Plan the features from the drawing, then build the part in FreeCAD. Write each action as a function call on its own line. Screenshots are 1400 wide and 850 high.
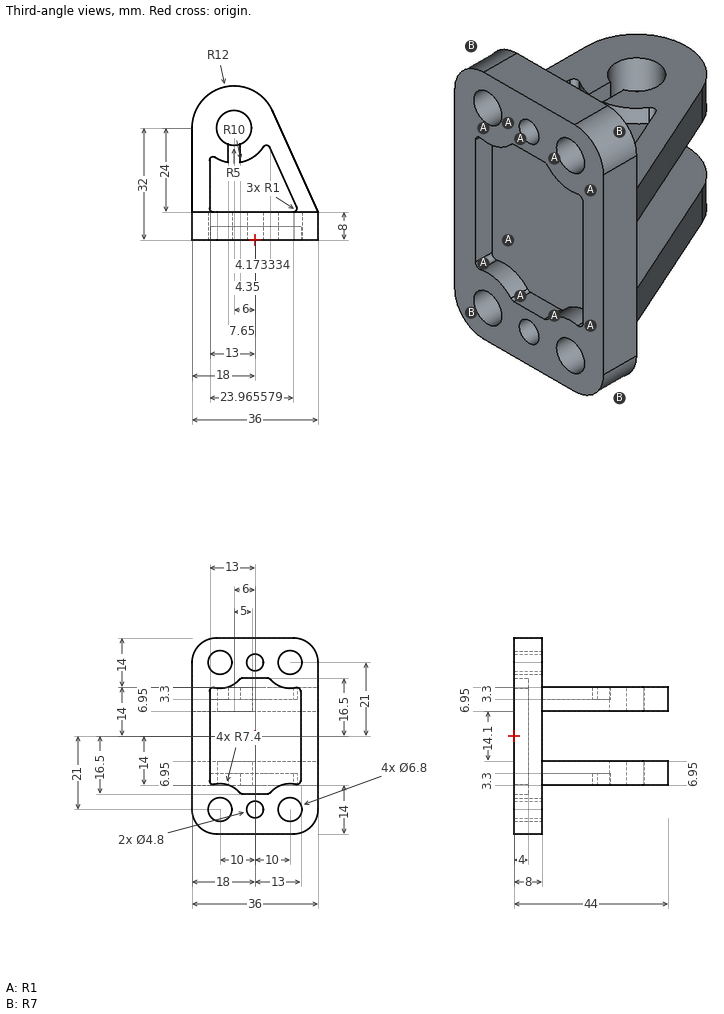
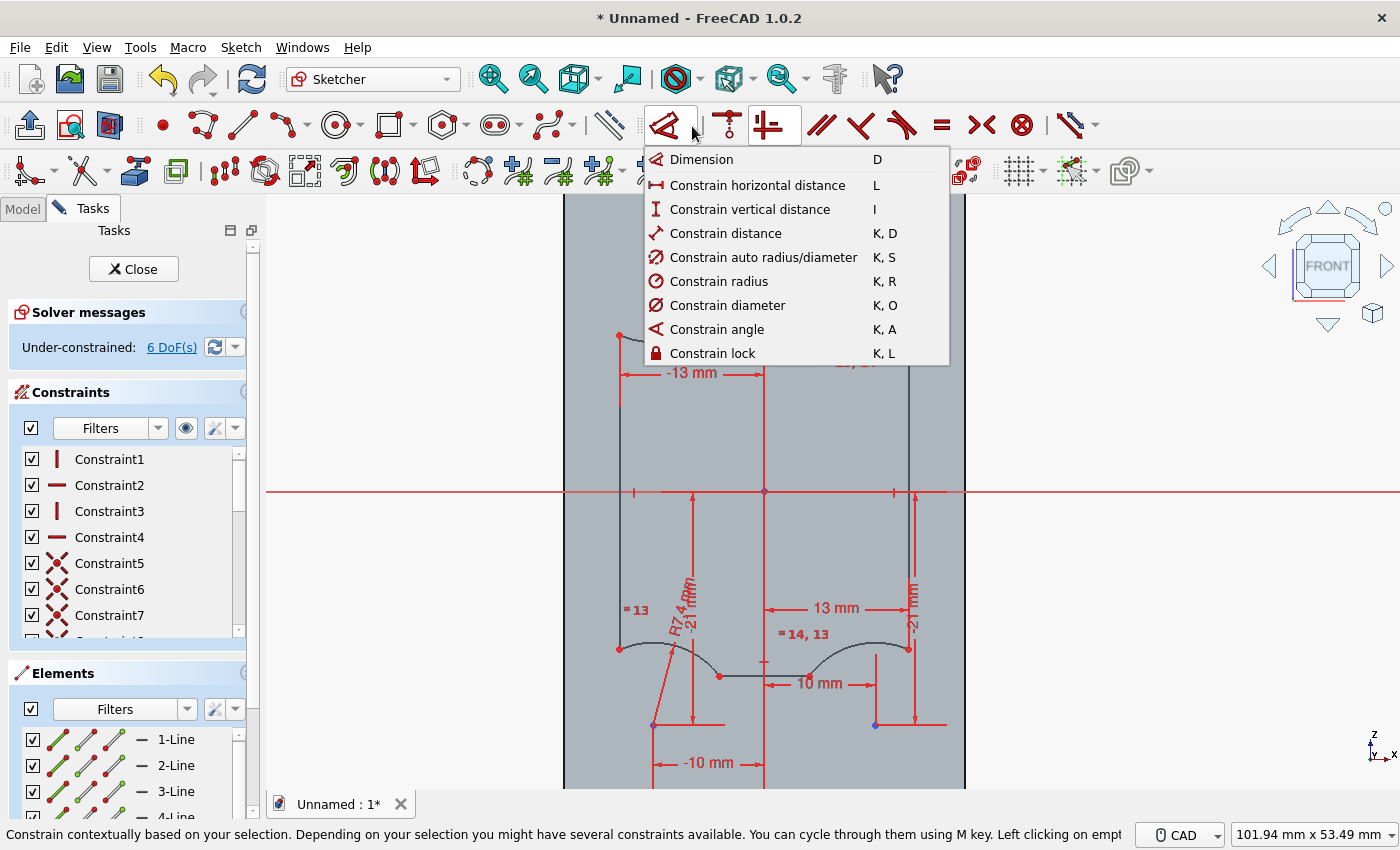
click(797, 185)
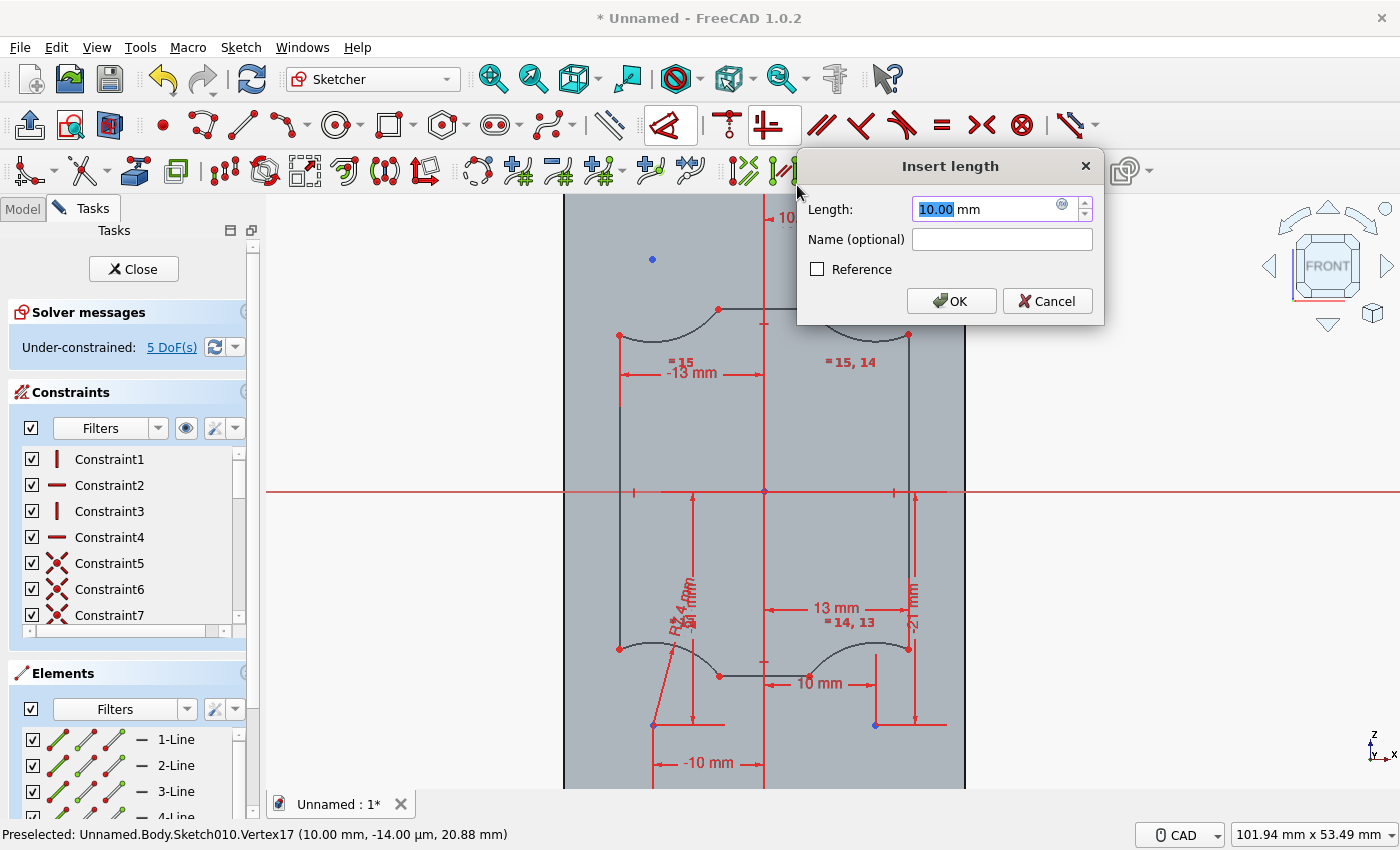
text(10)
key(Return)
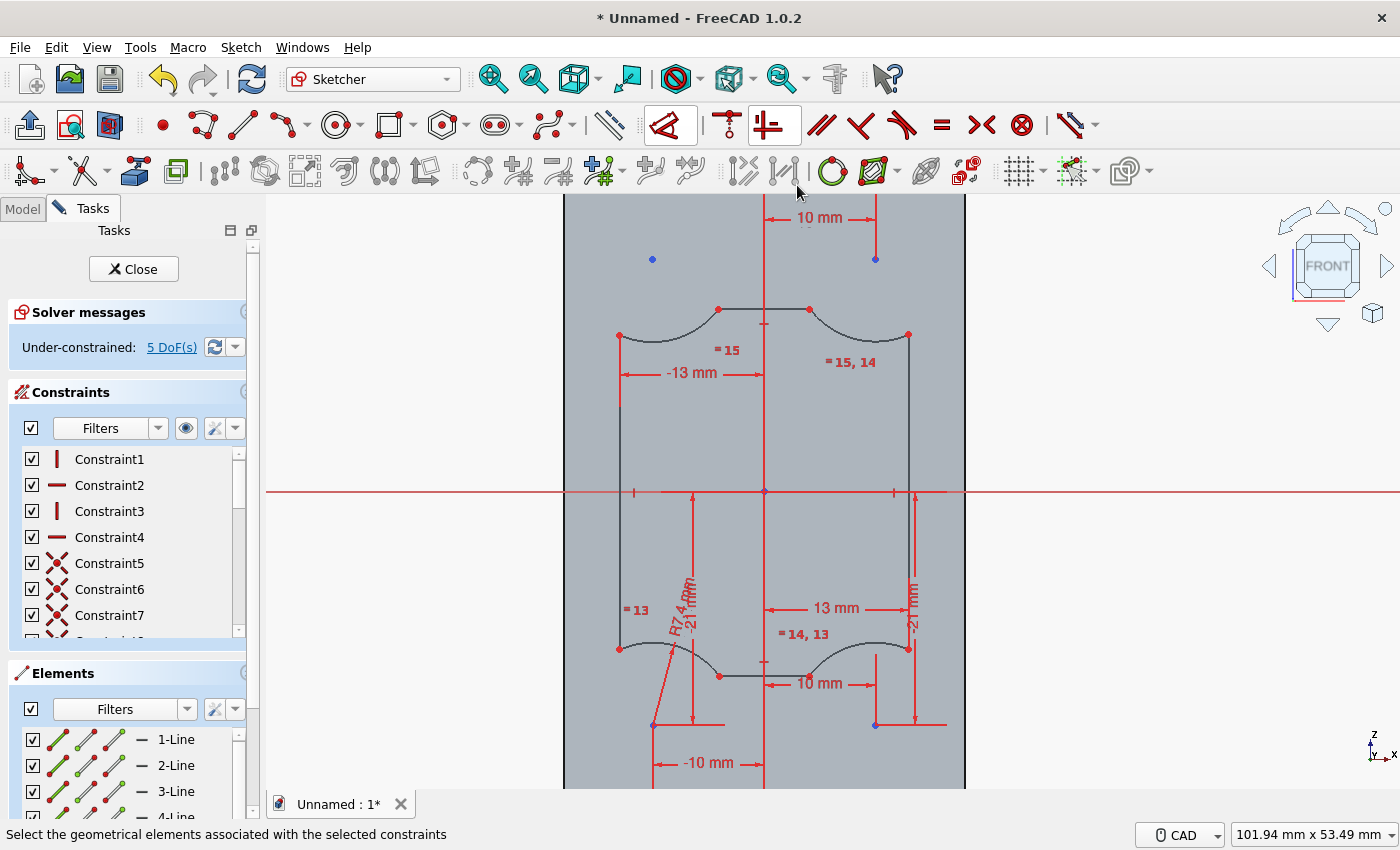
click(876, 259)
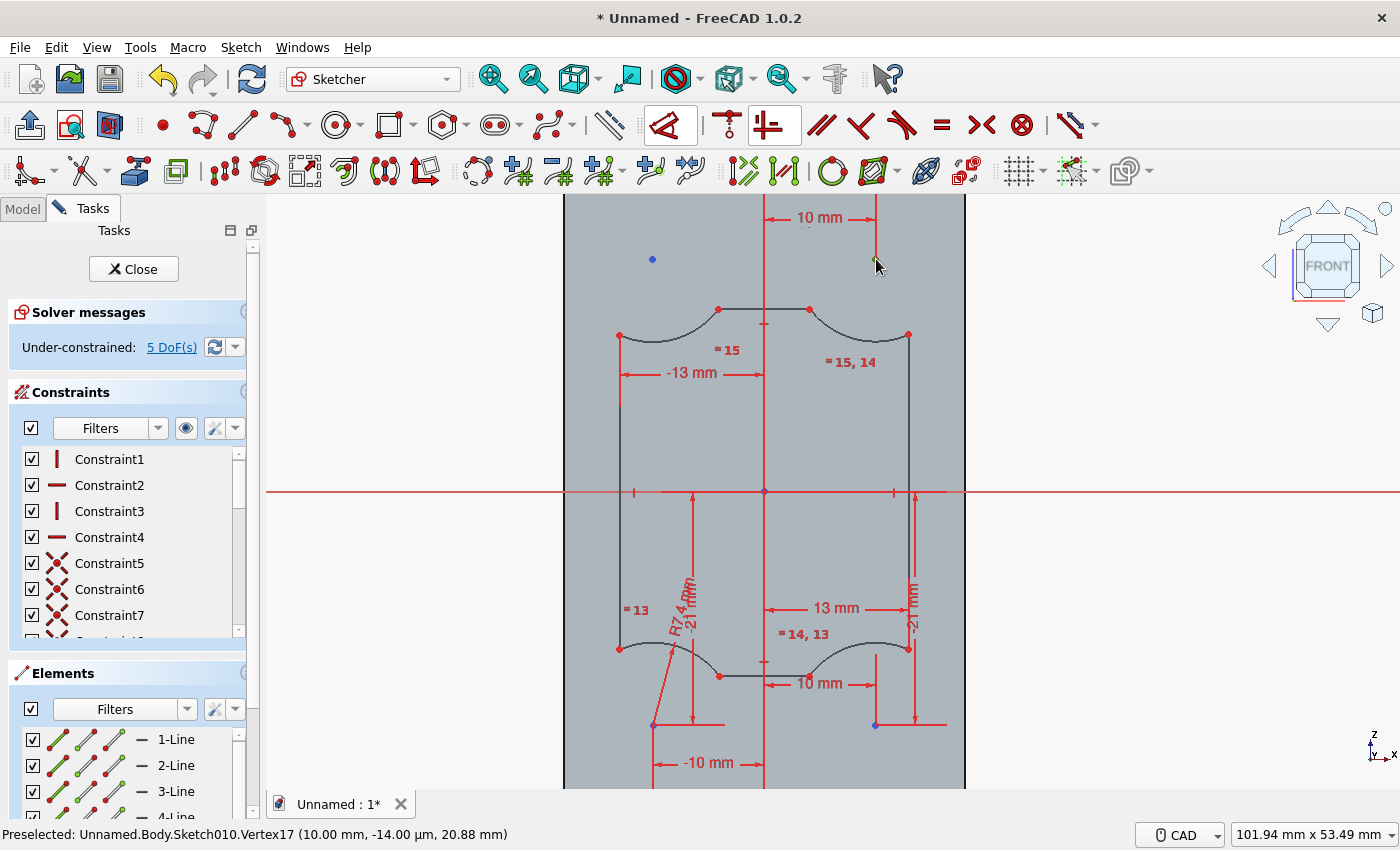
key(i)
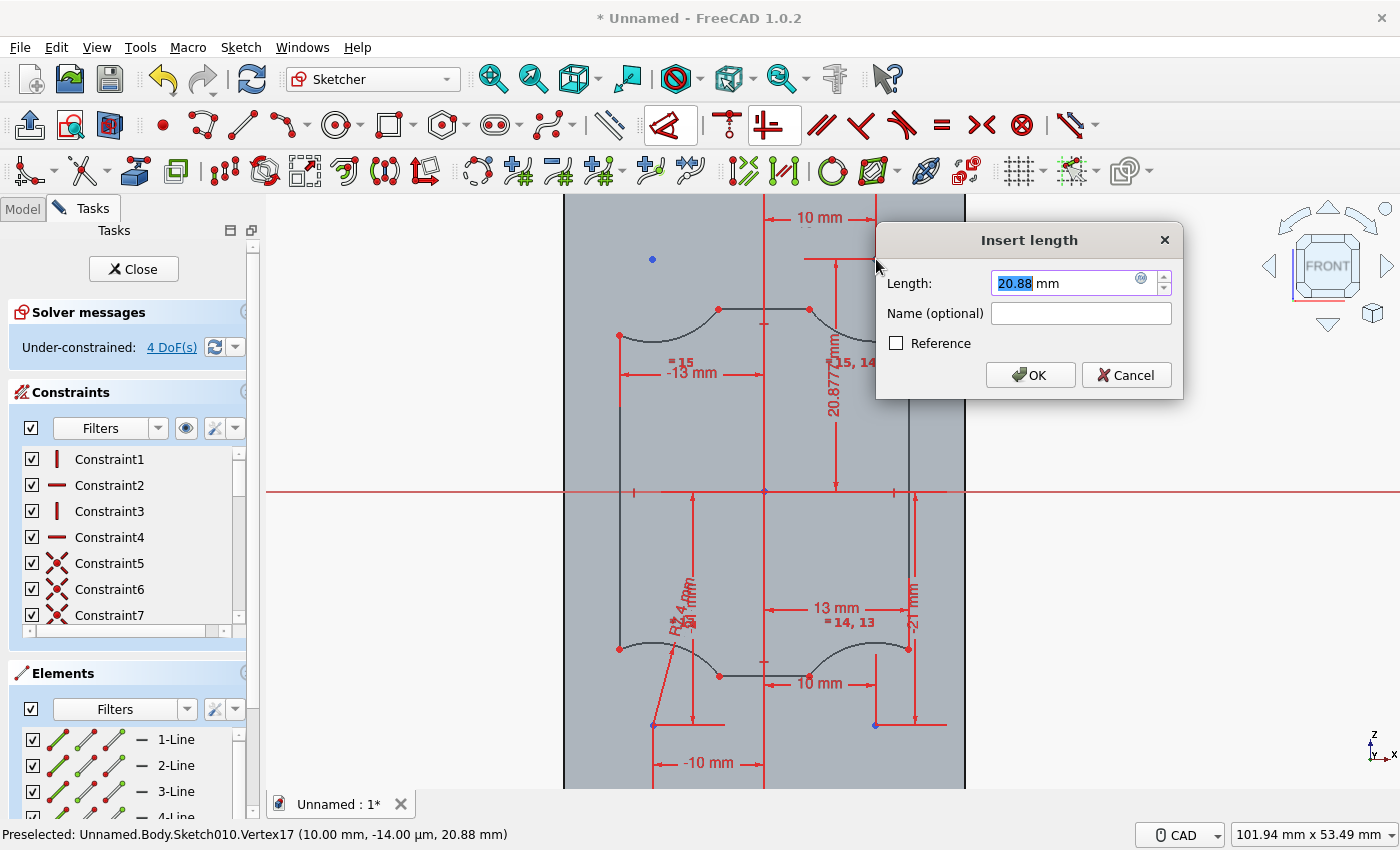
text(21)
key(Return)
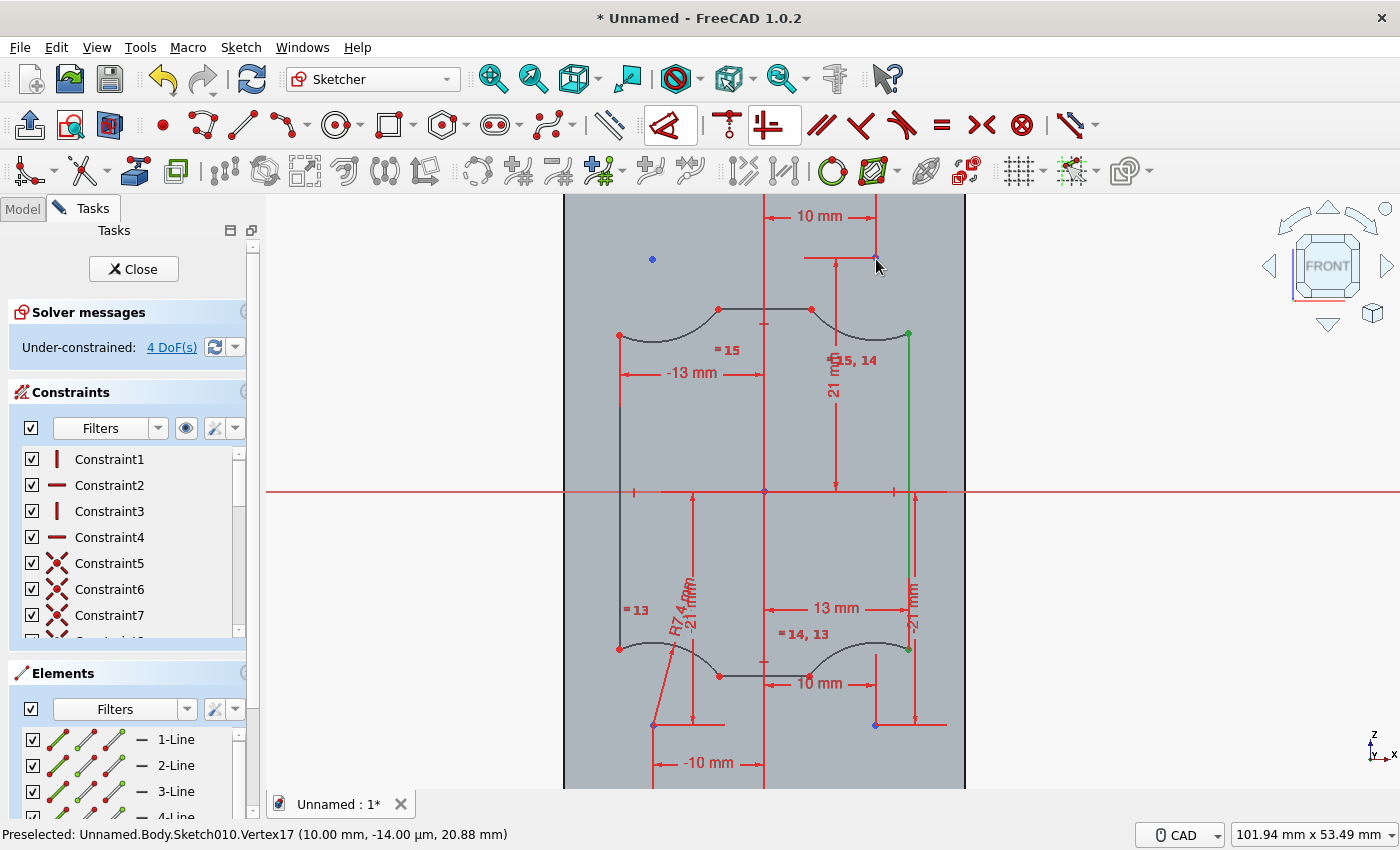
click(653, 260)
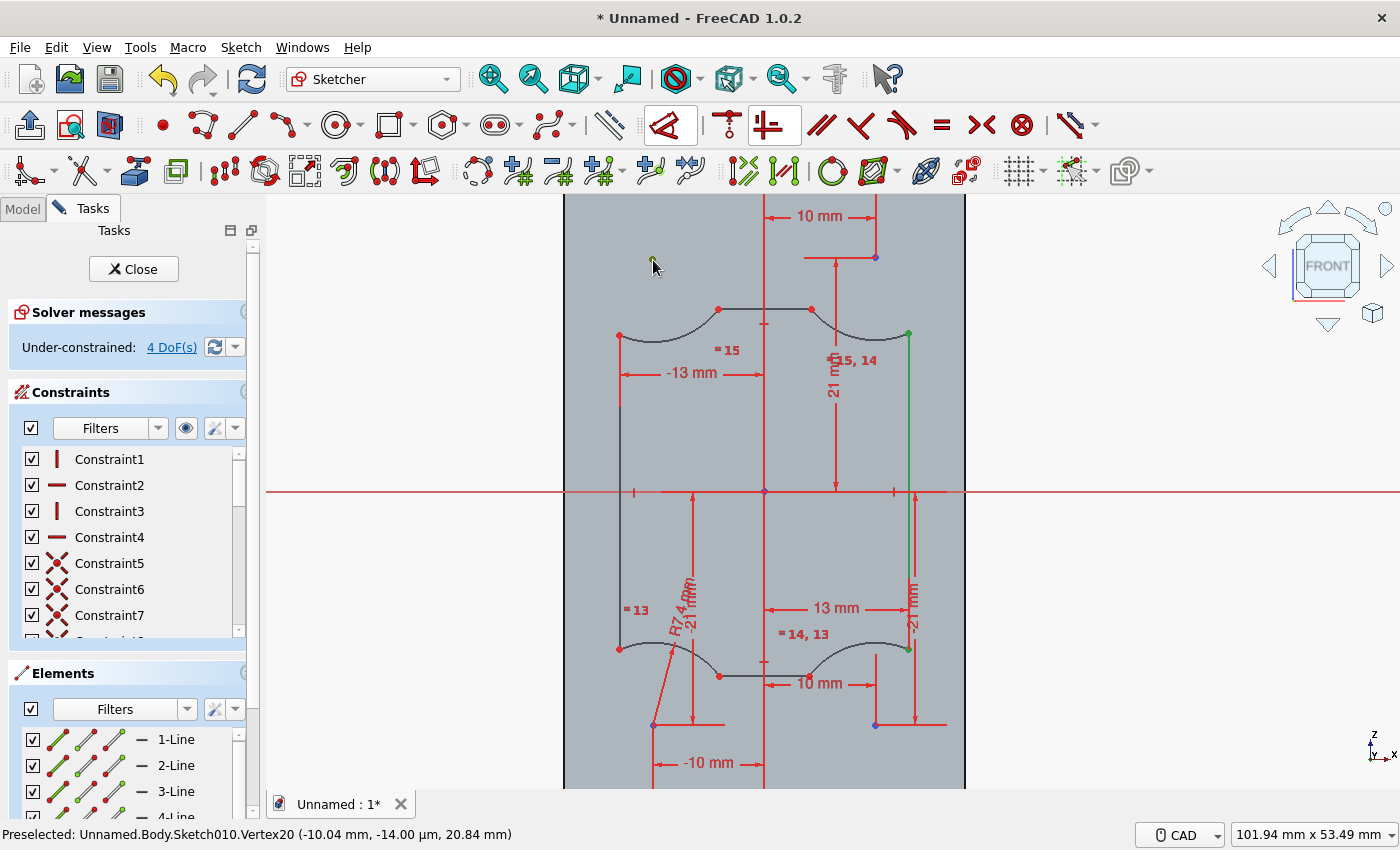
key(l)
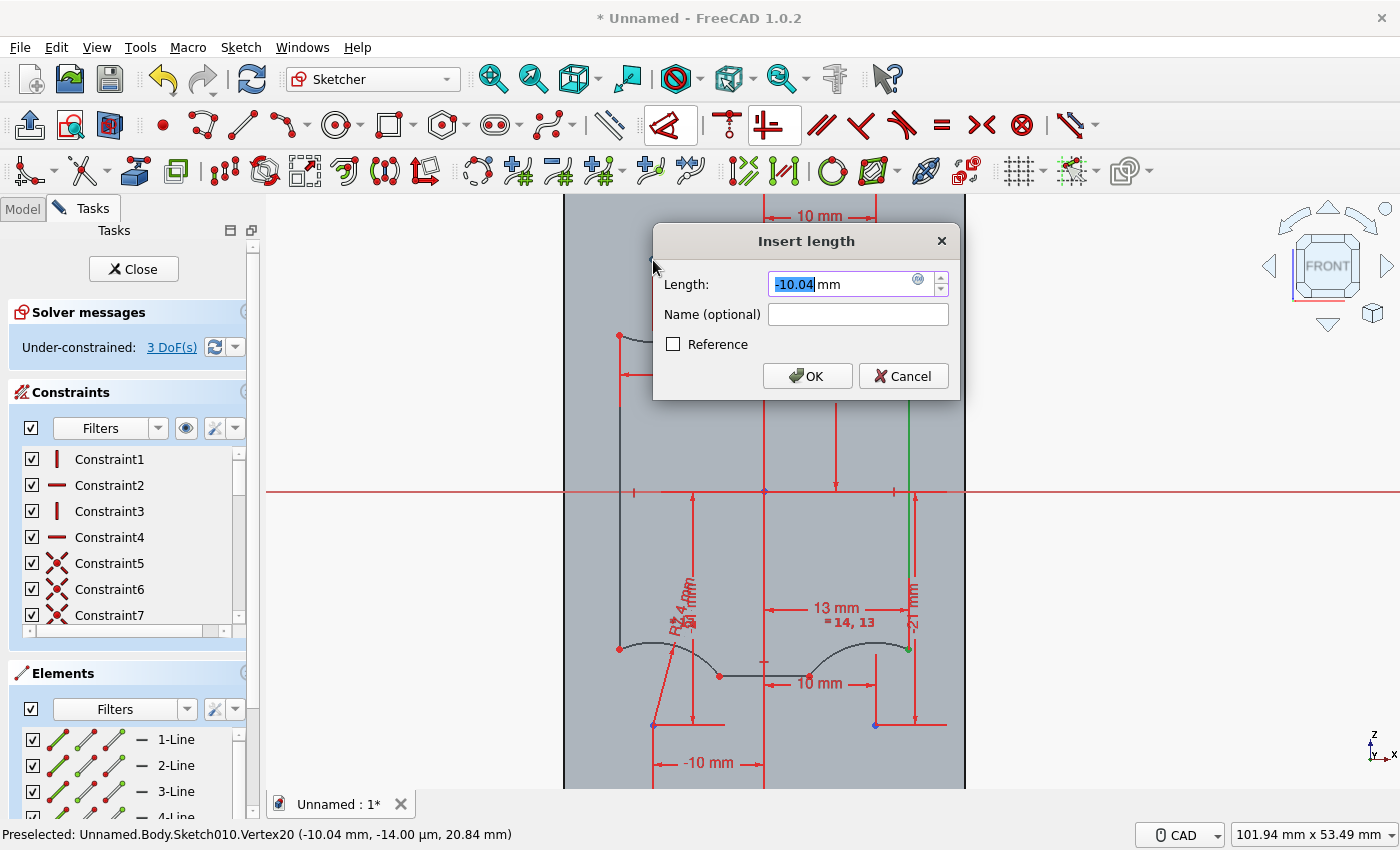
text(-10)
key(Return)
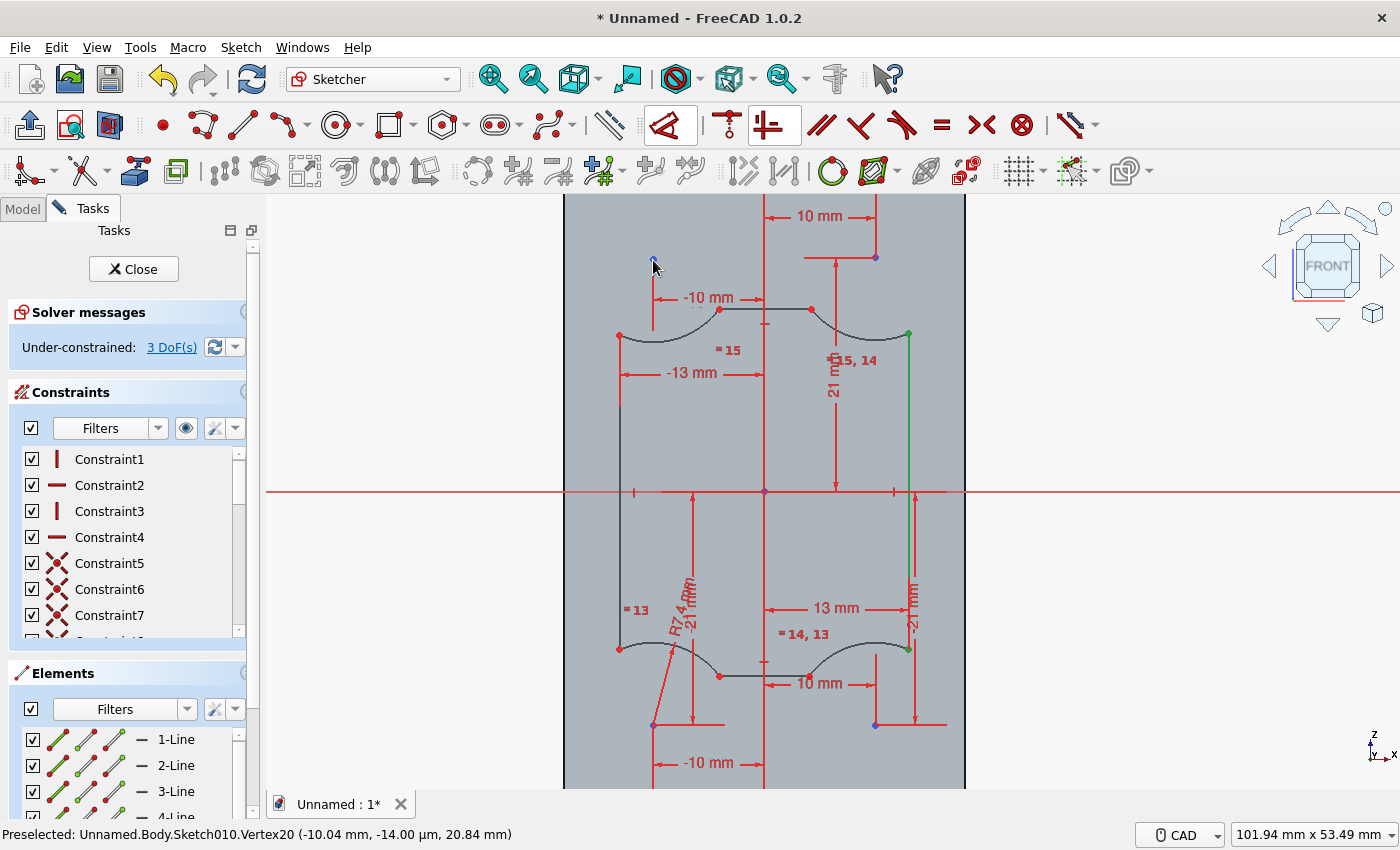
click(653, 260)